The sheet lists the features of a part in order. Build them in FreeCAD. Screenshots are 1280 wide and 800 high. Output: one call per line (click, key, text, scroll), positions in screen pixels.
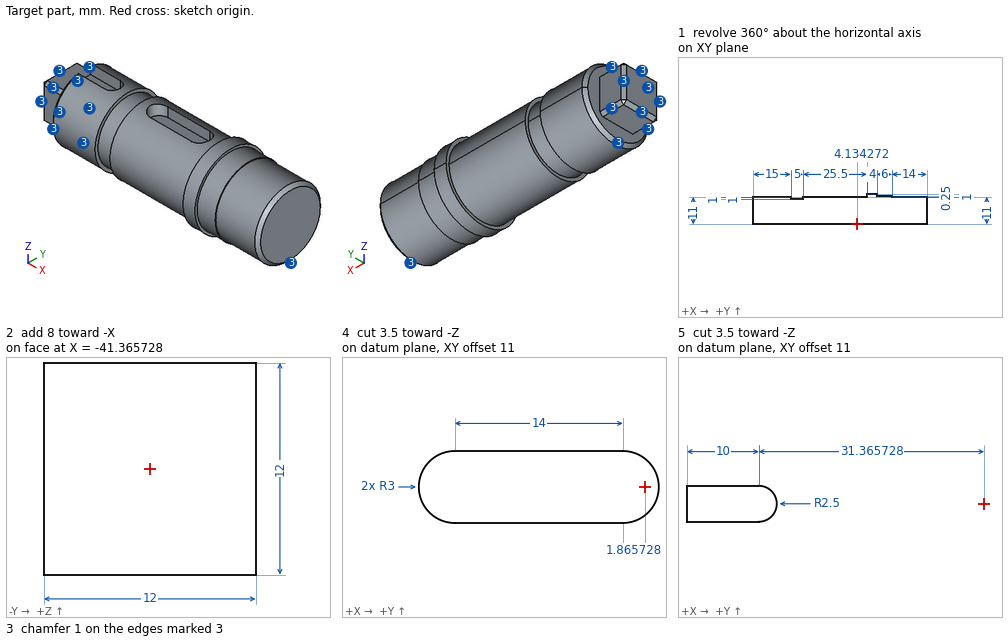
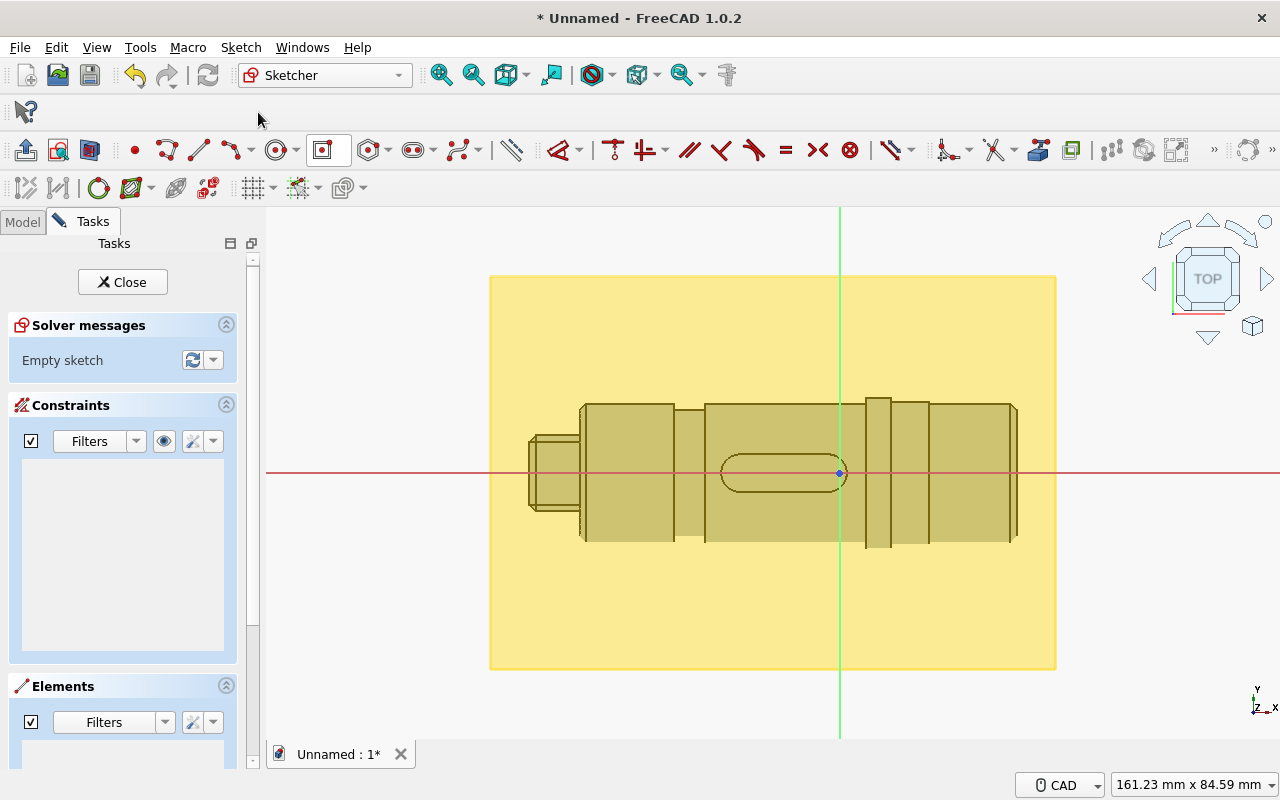
scroll(606, 473, up, 10)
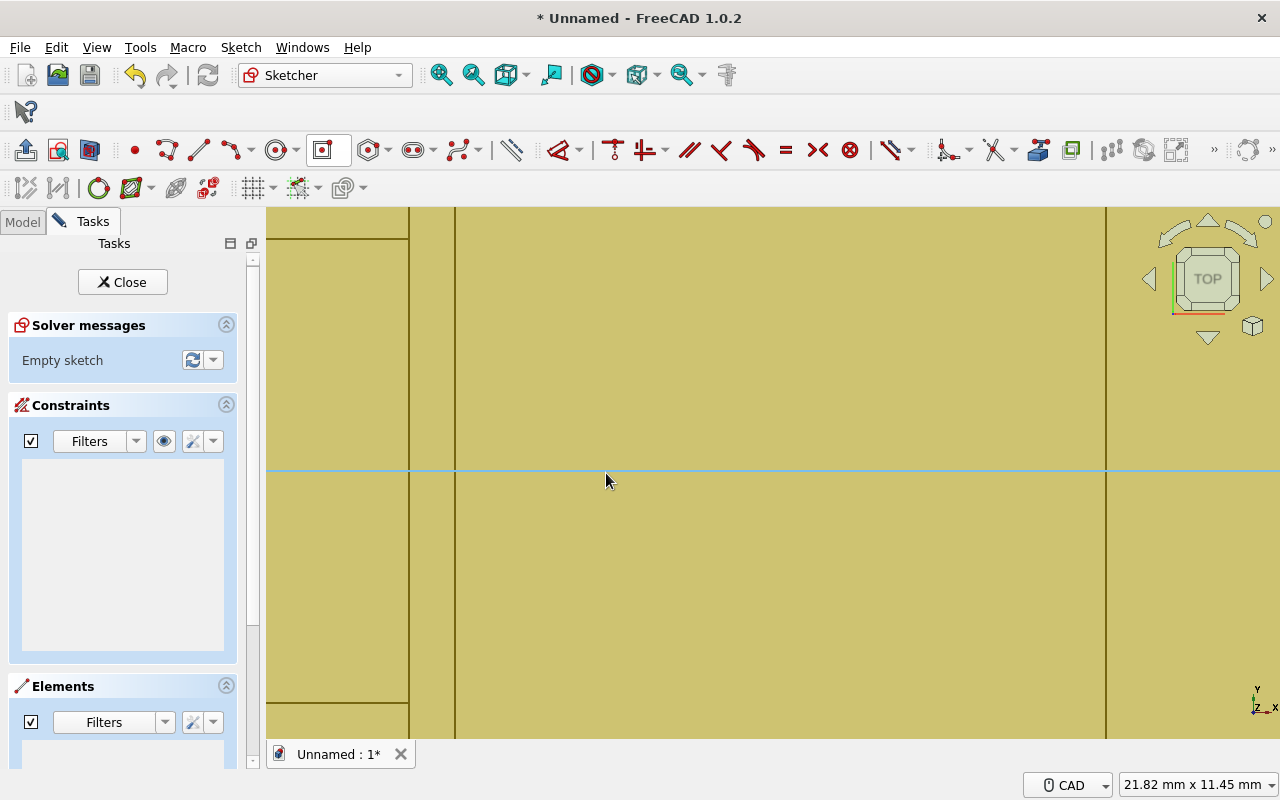
click(168, 150)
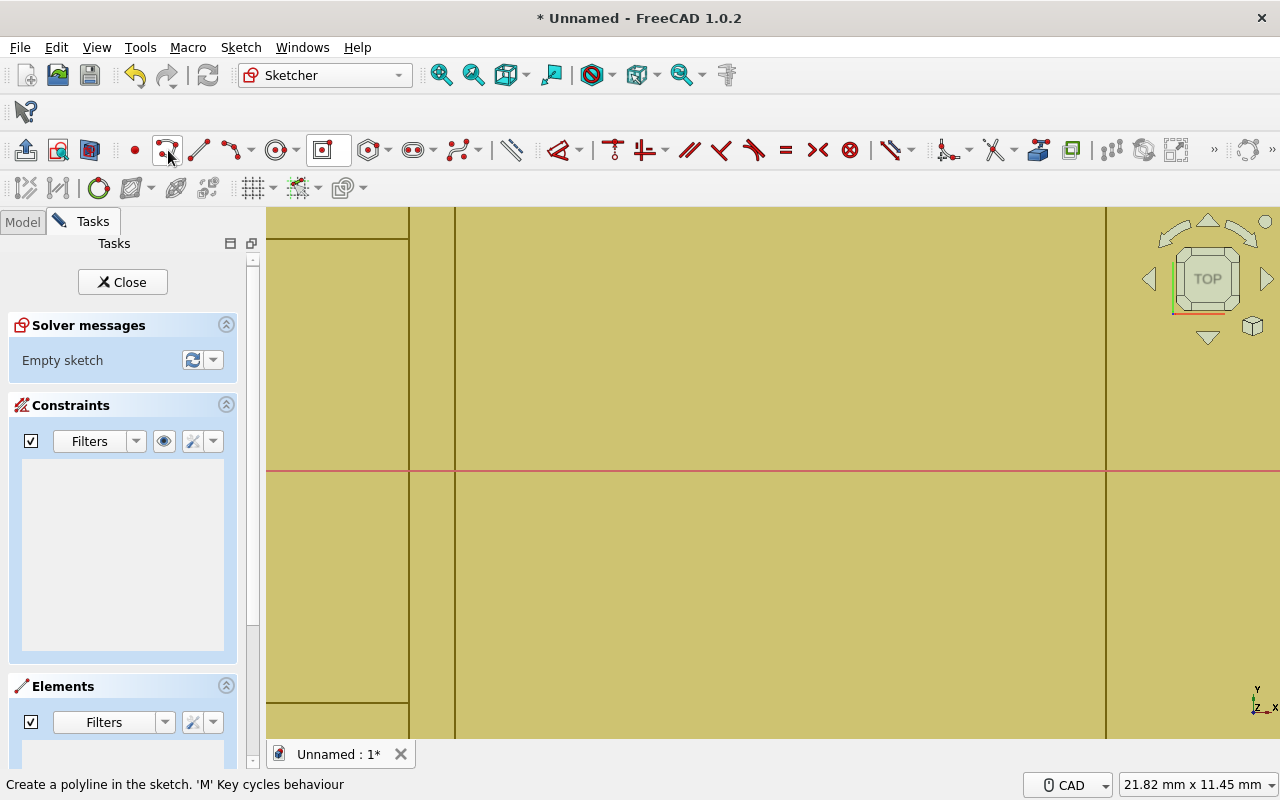
click(874, 355)
click(409, 355)
click(409, 587)
click(874, 587)
right_click(874, 587)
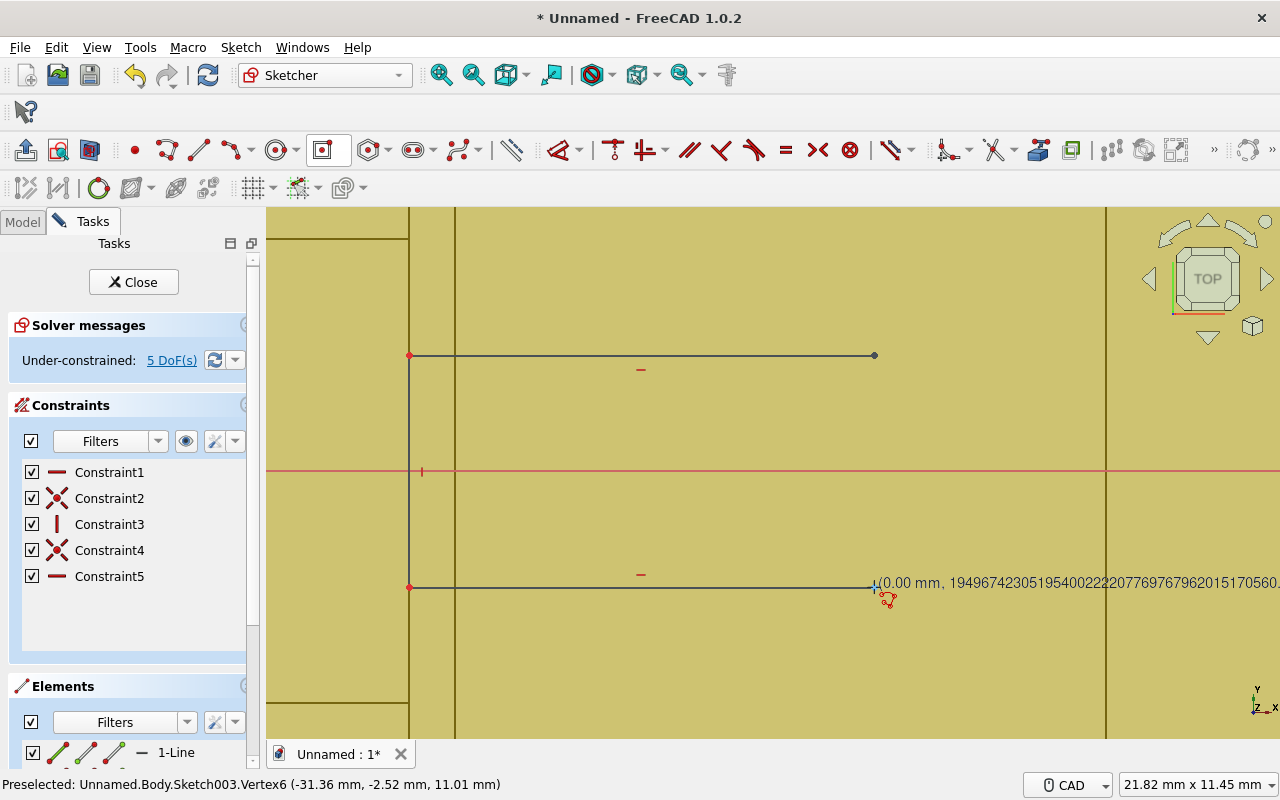
click(232, 150)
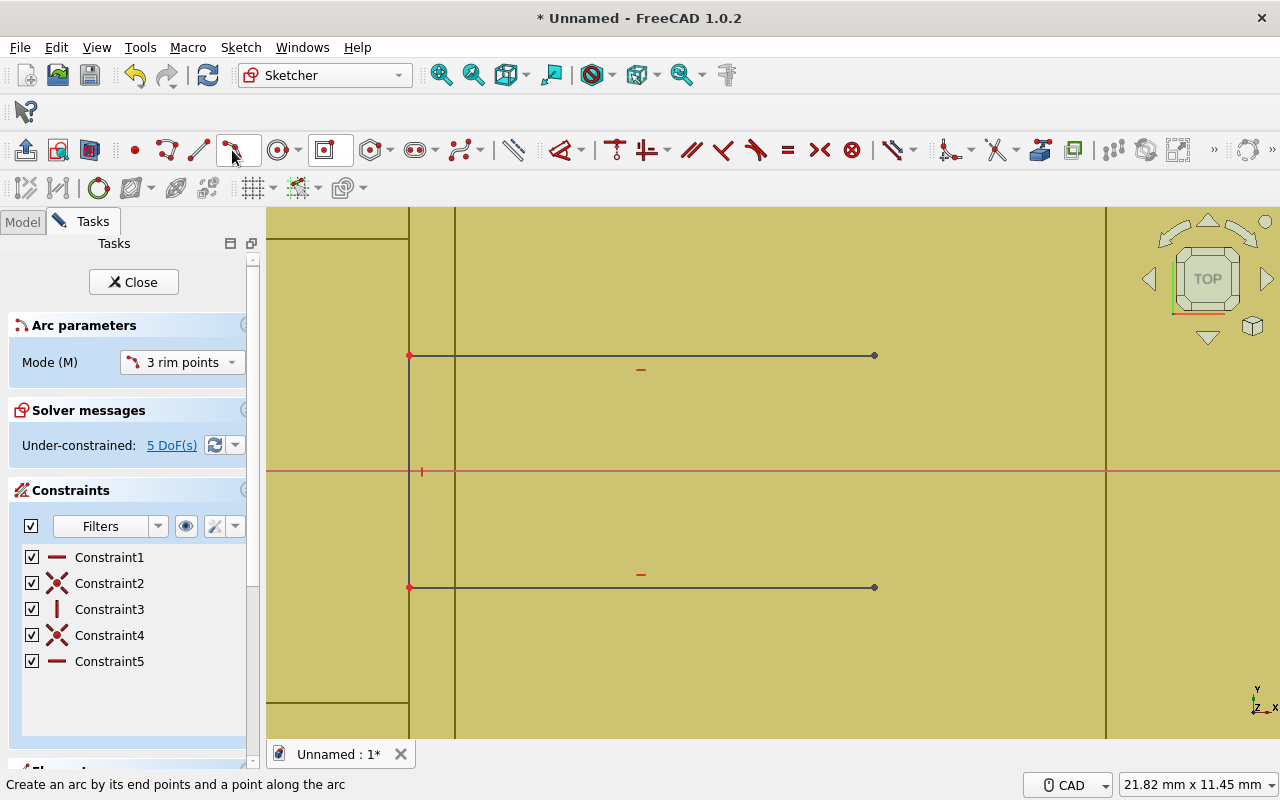
click(874, 588)
click(874, 356)
click(984, 507)
key(Escape)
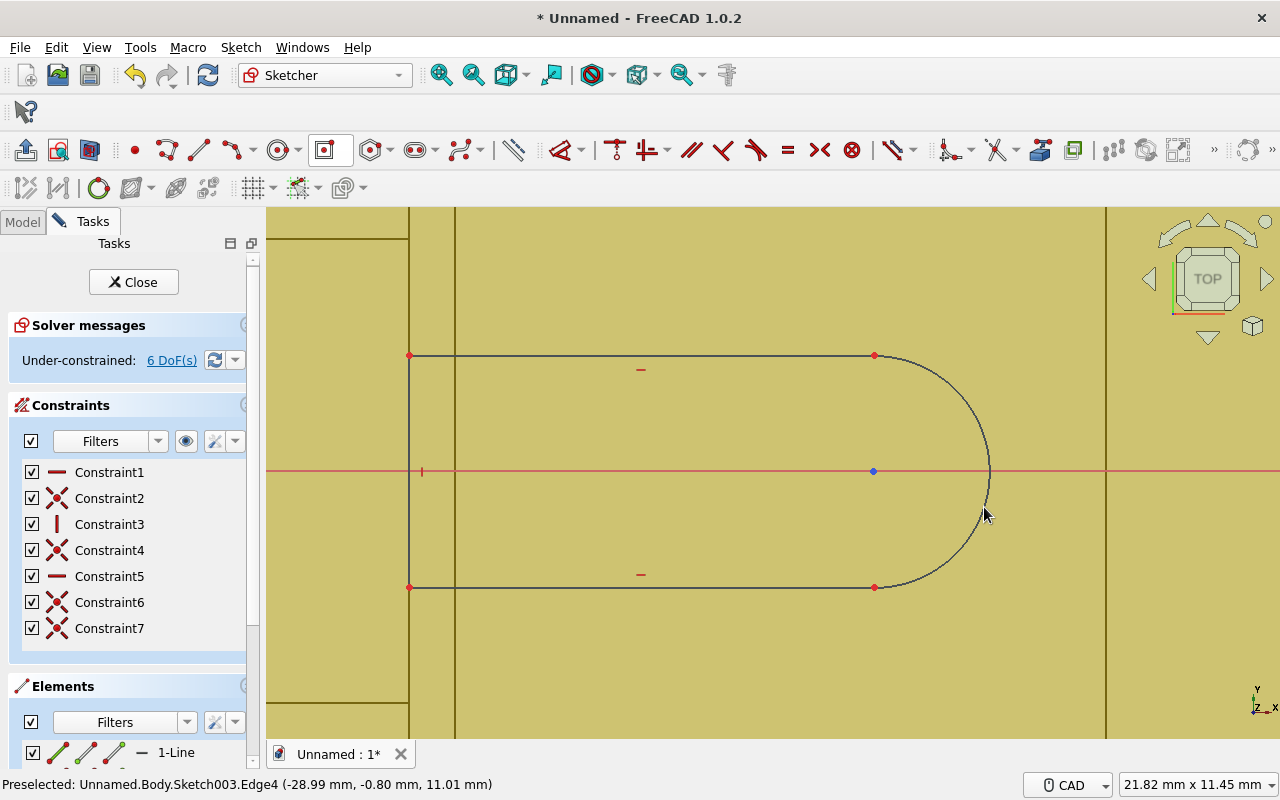
click(735, 356)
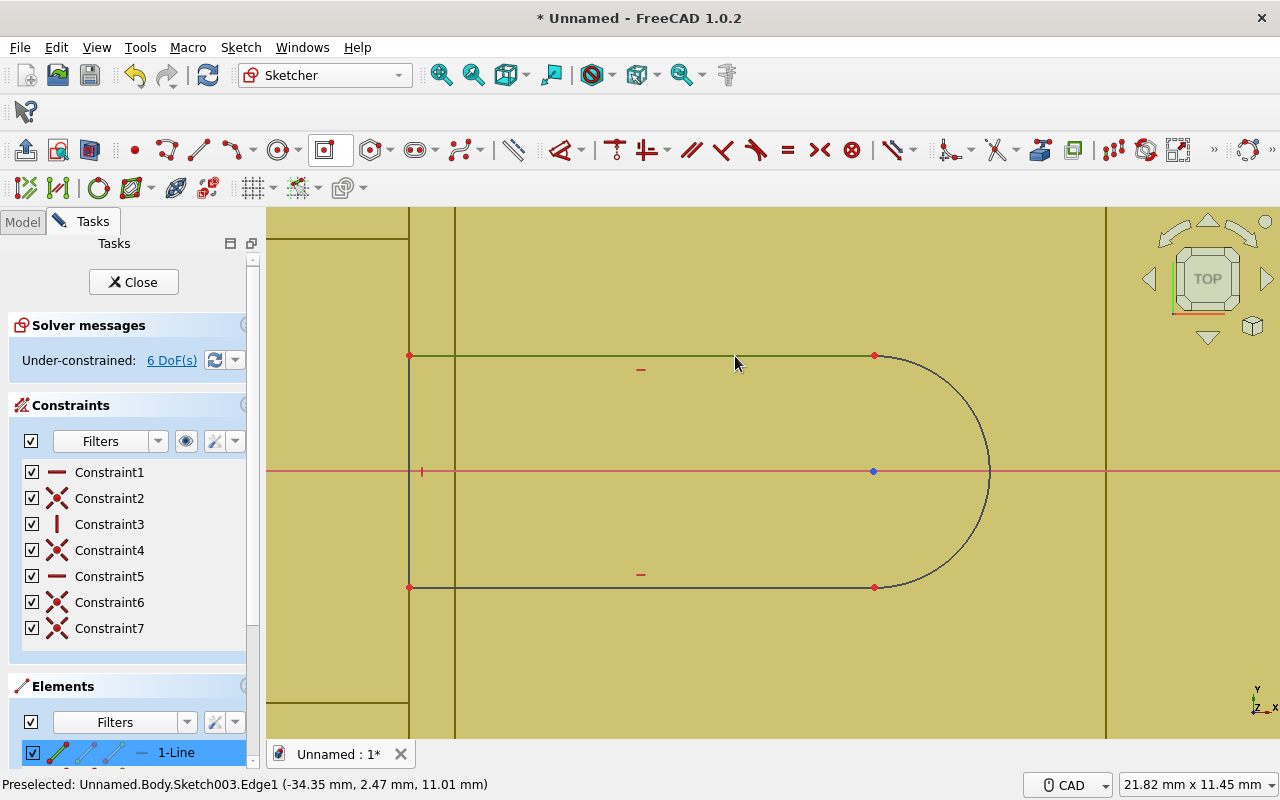
click(968, 540)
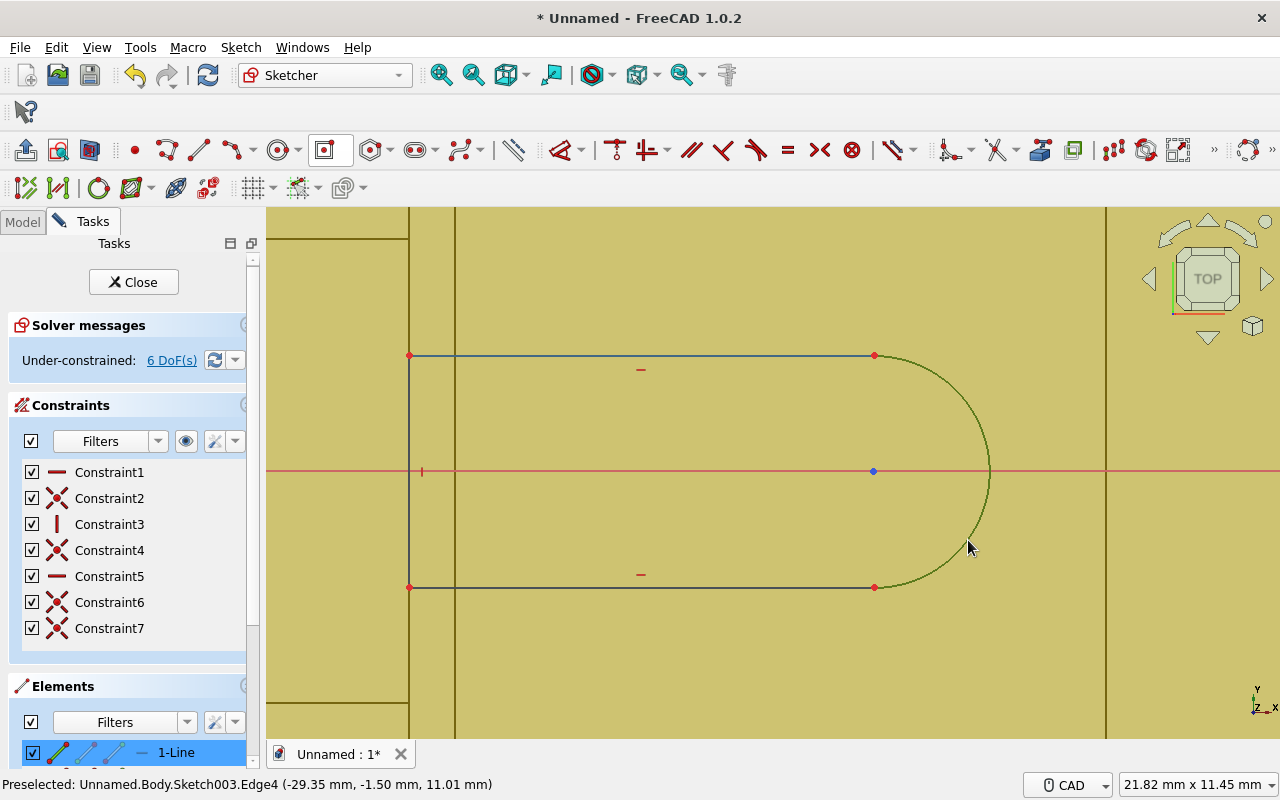
click(756, 150)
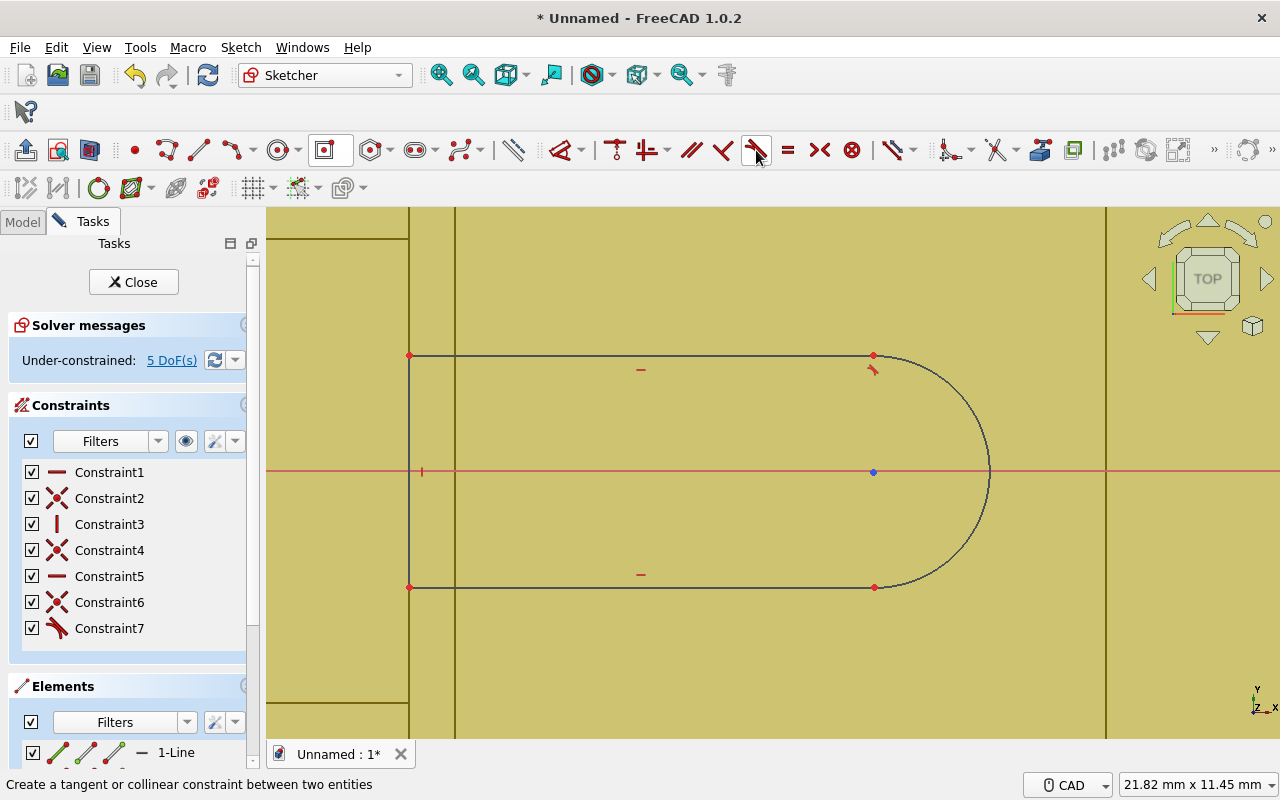
click(548, 588)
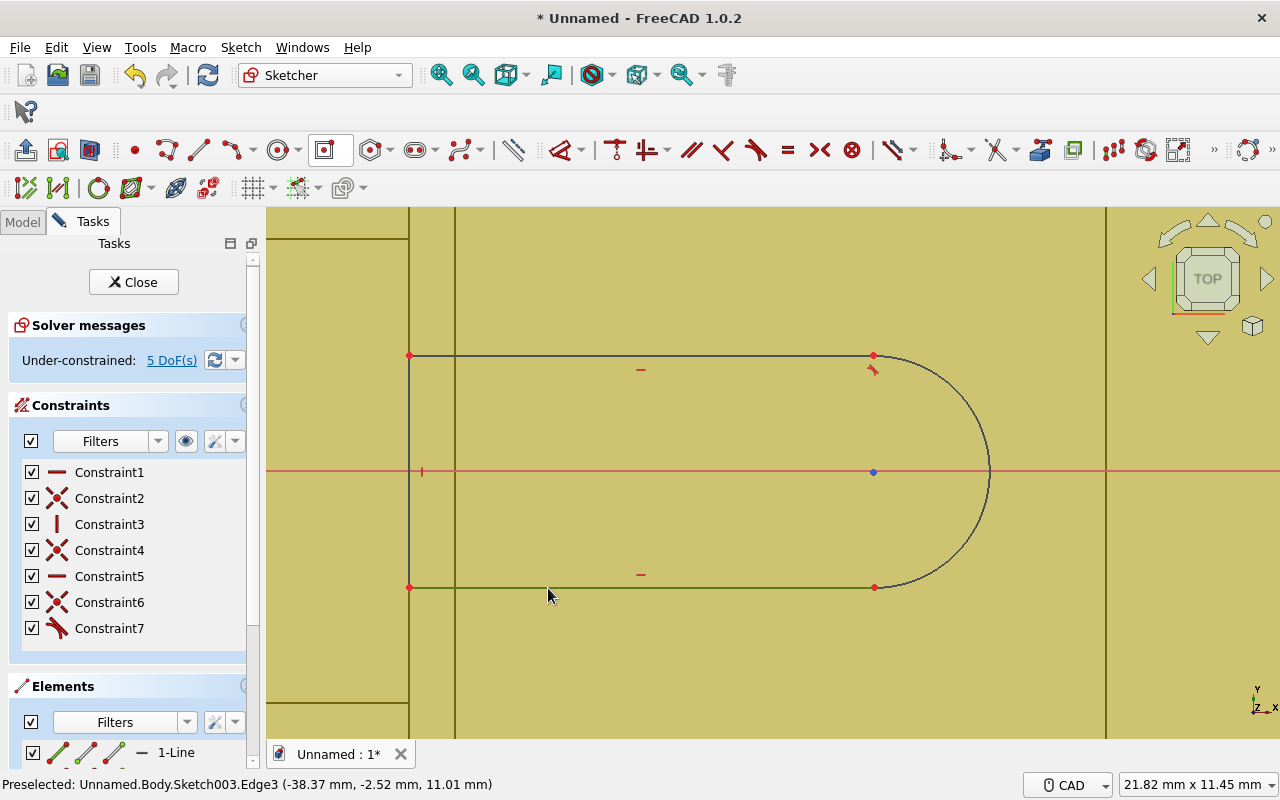
click(968, 540)